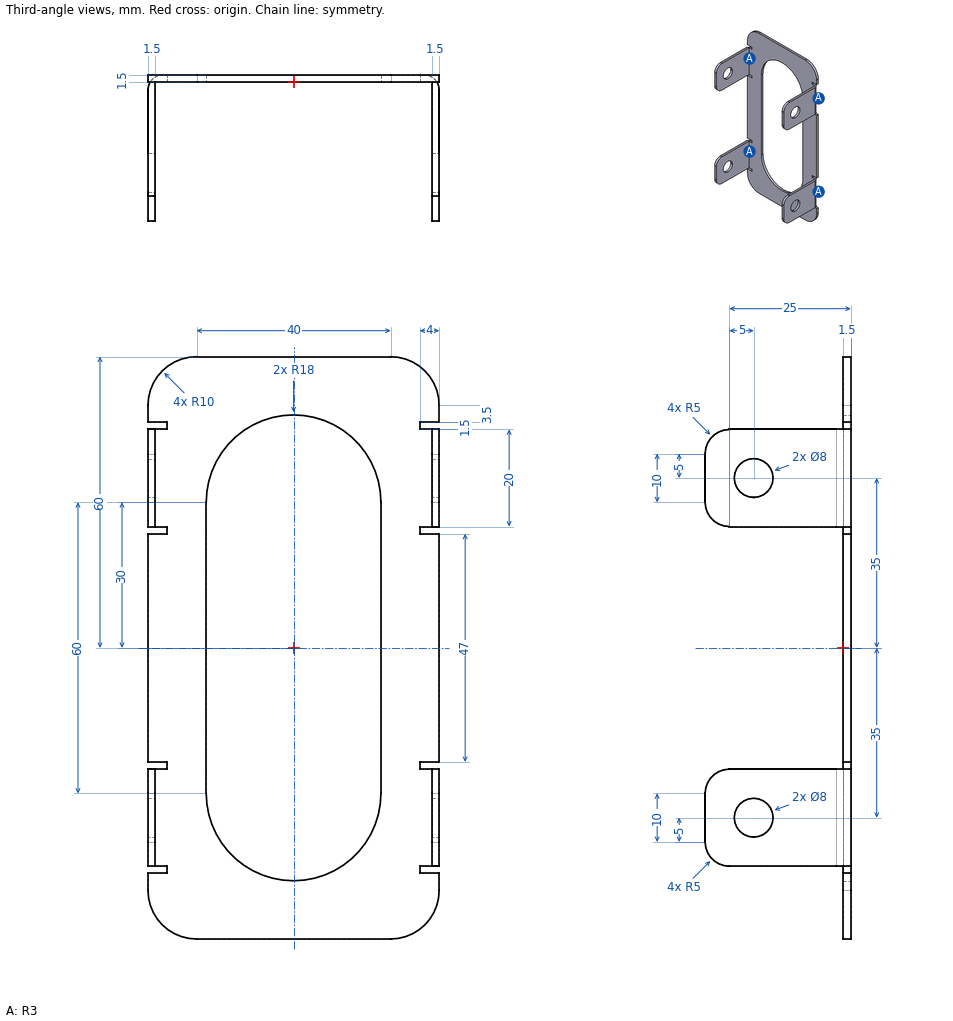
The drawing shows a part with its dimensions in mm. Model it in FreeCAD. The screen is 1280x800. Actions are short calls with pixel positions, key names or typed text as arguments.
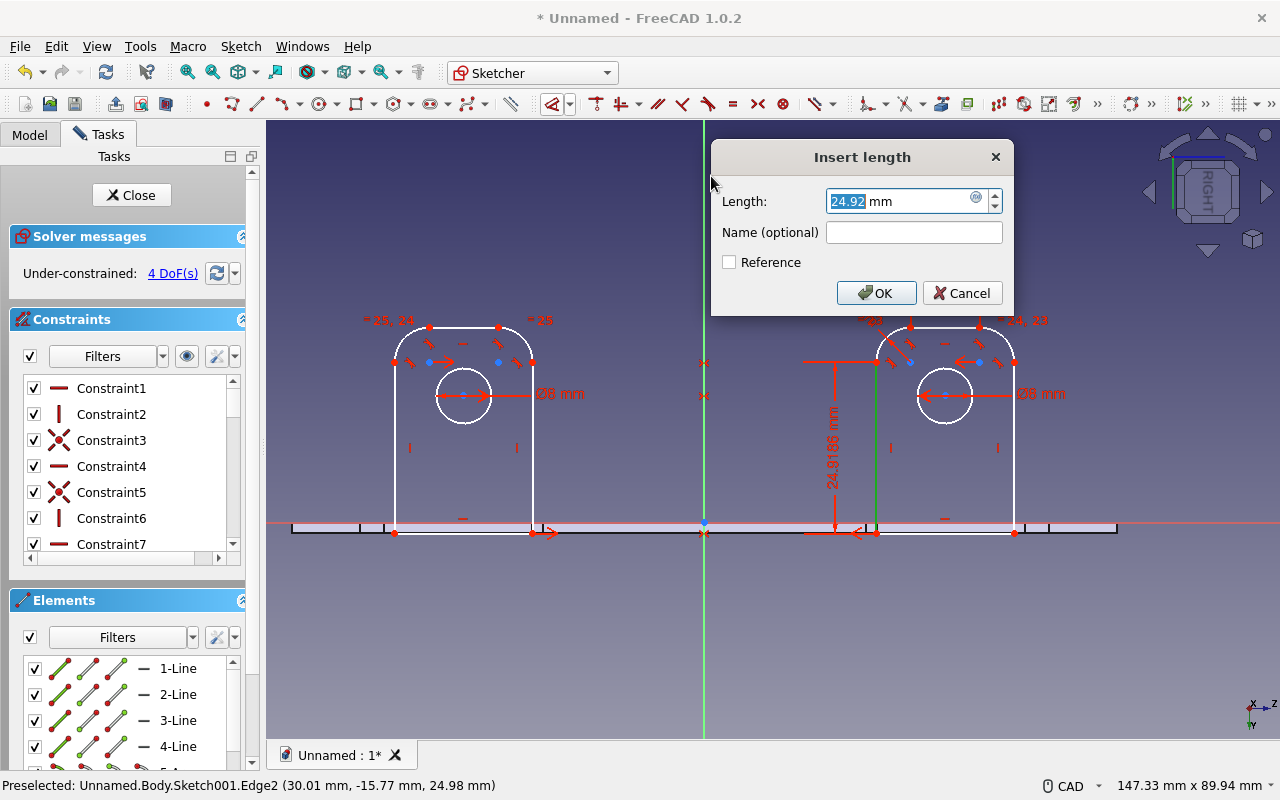
text(25)
key(Return)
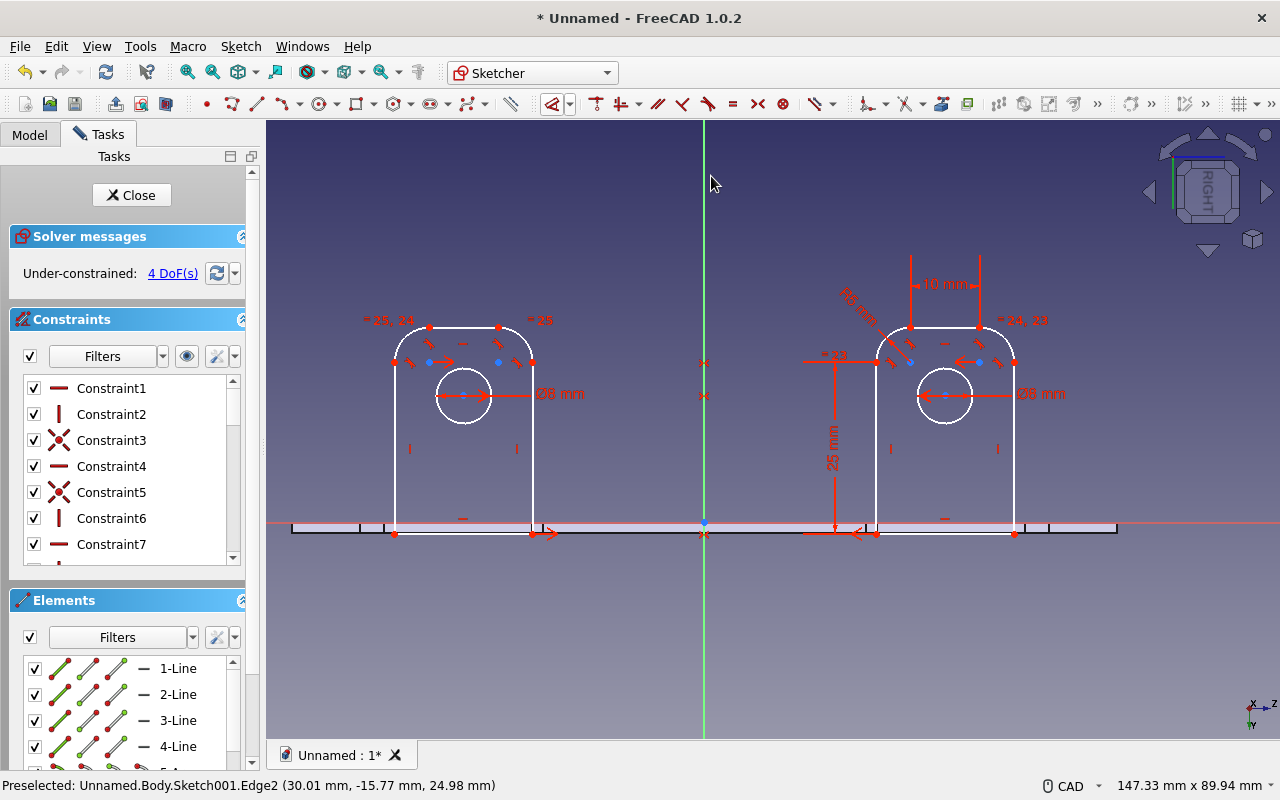
click(945, 396)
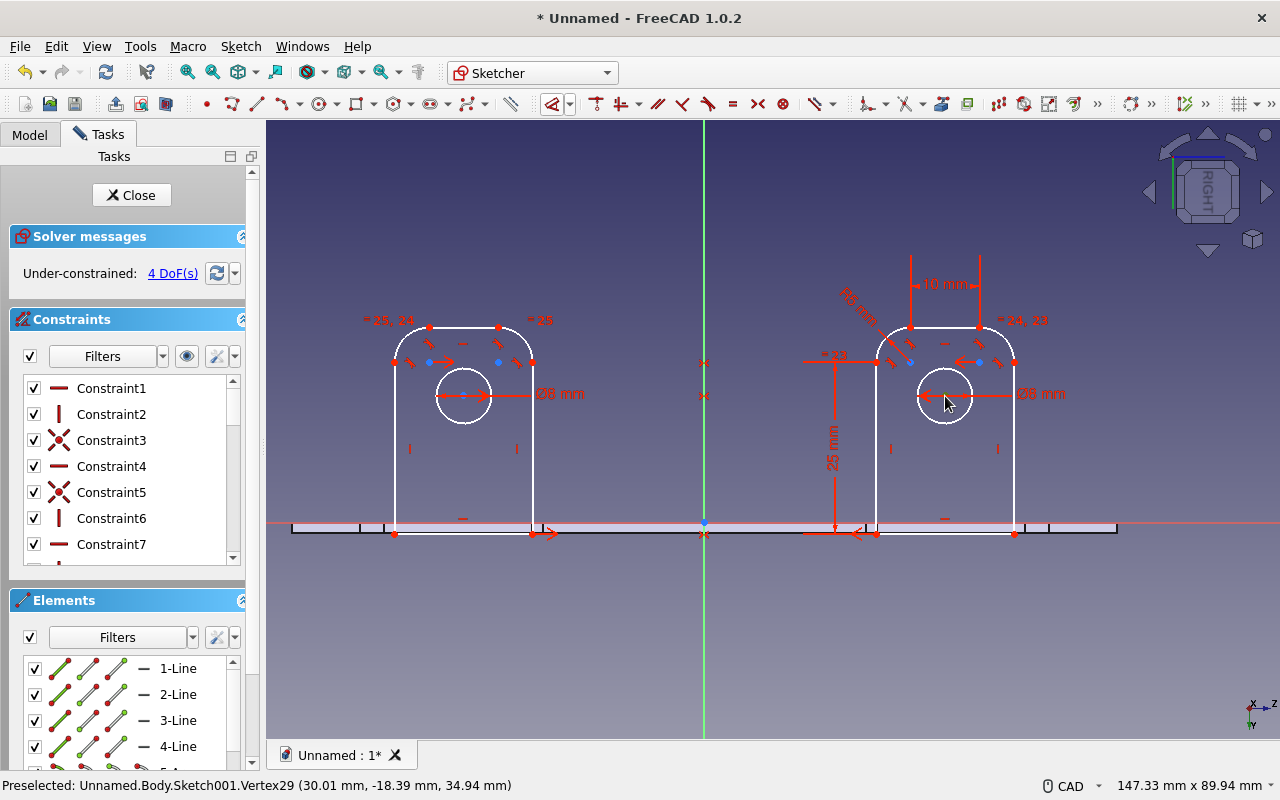
key(l)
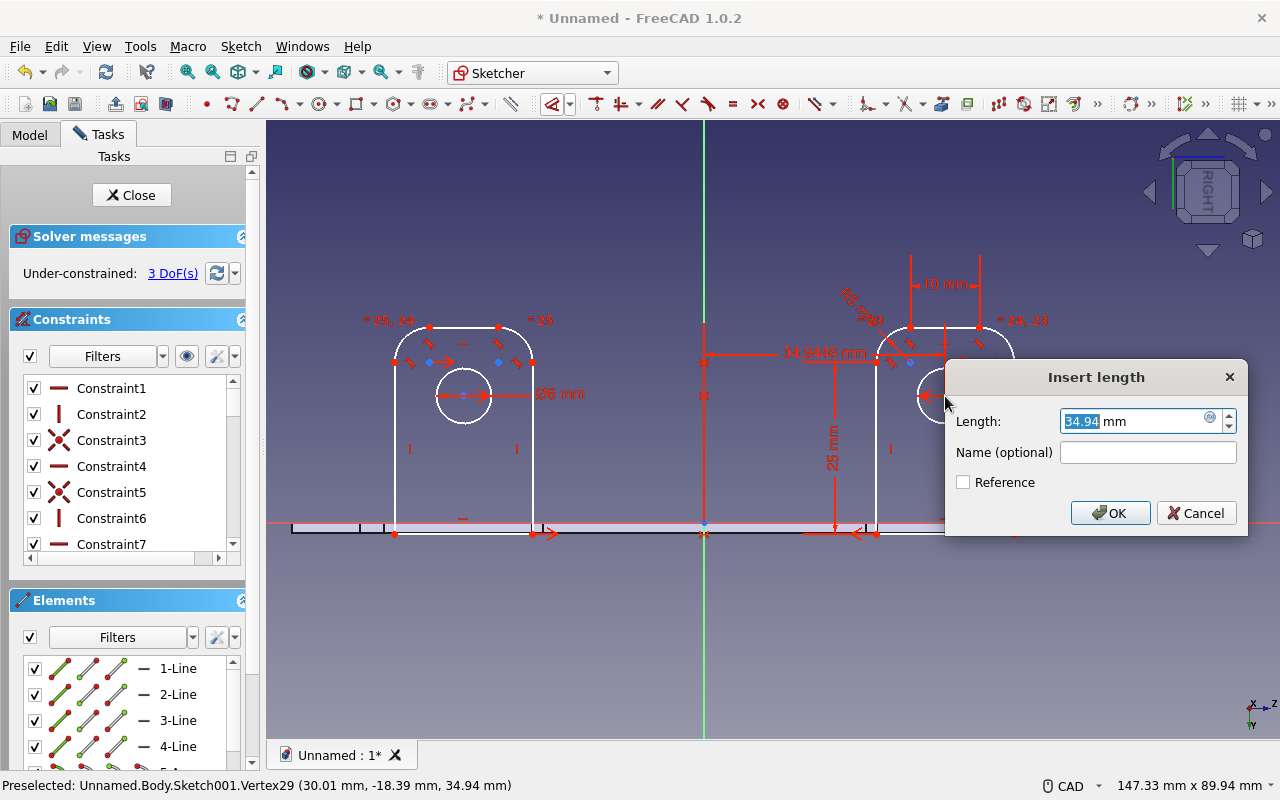
text(35)
key(Return)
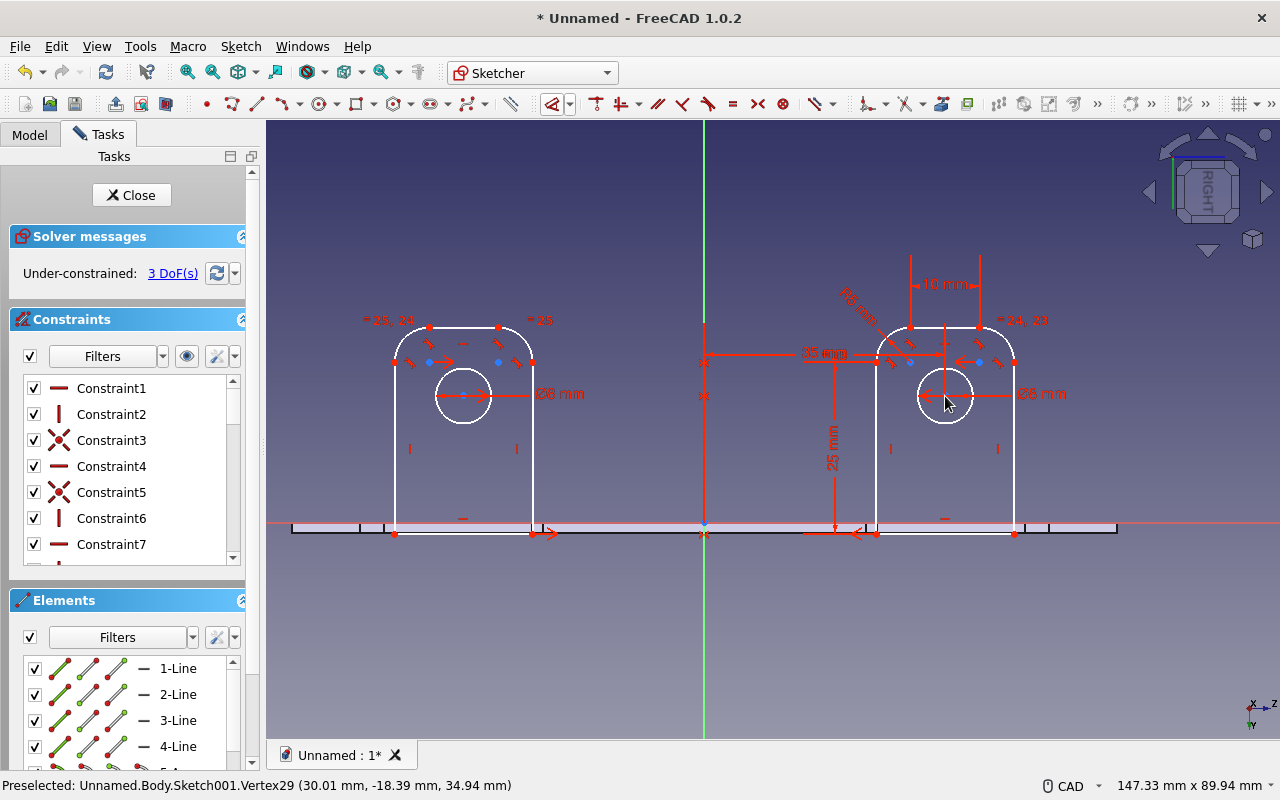
click(980, 328)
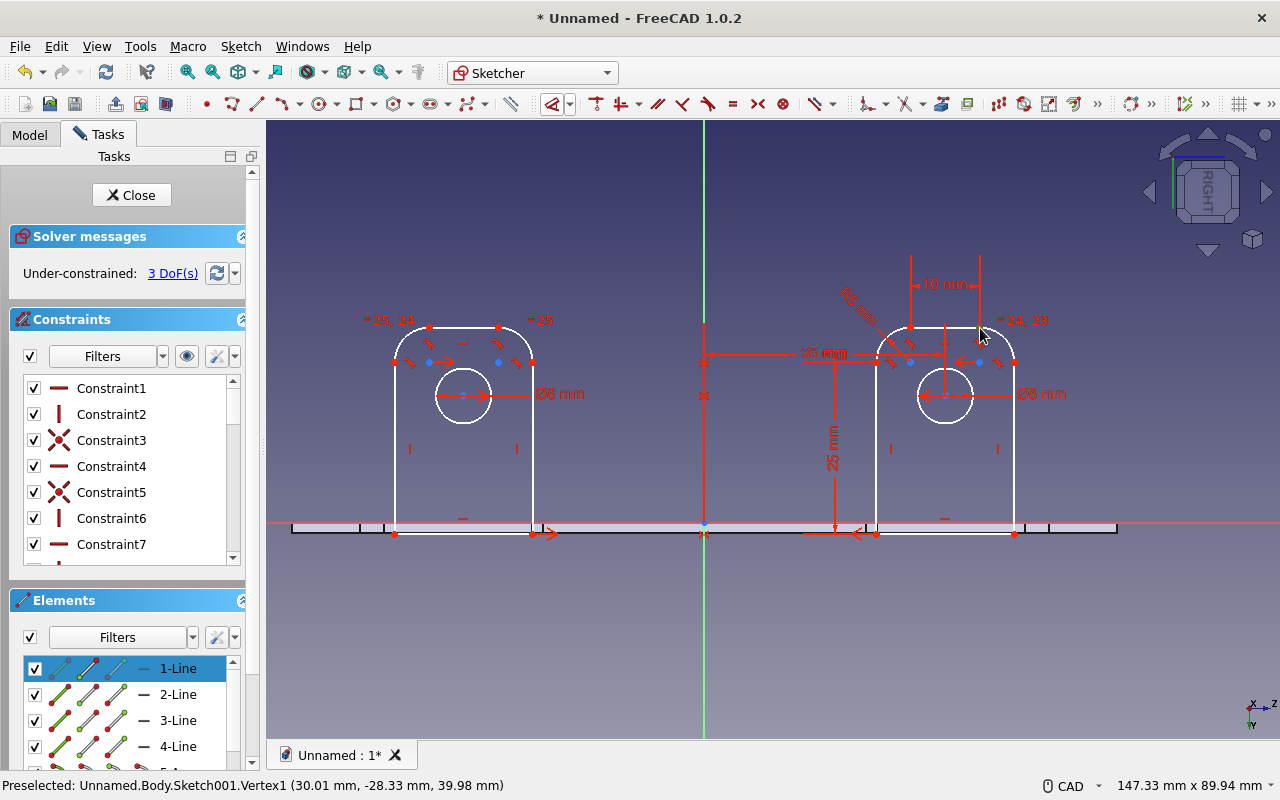
click(945, 396)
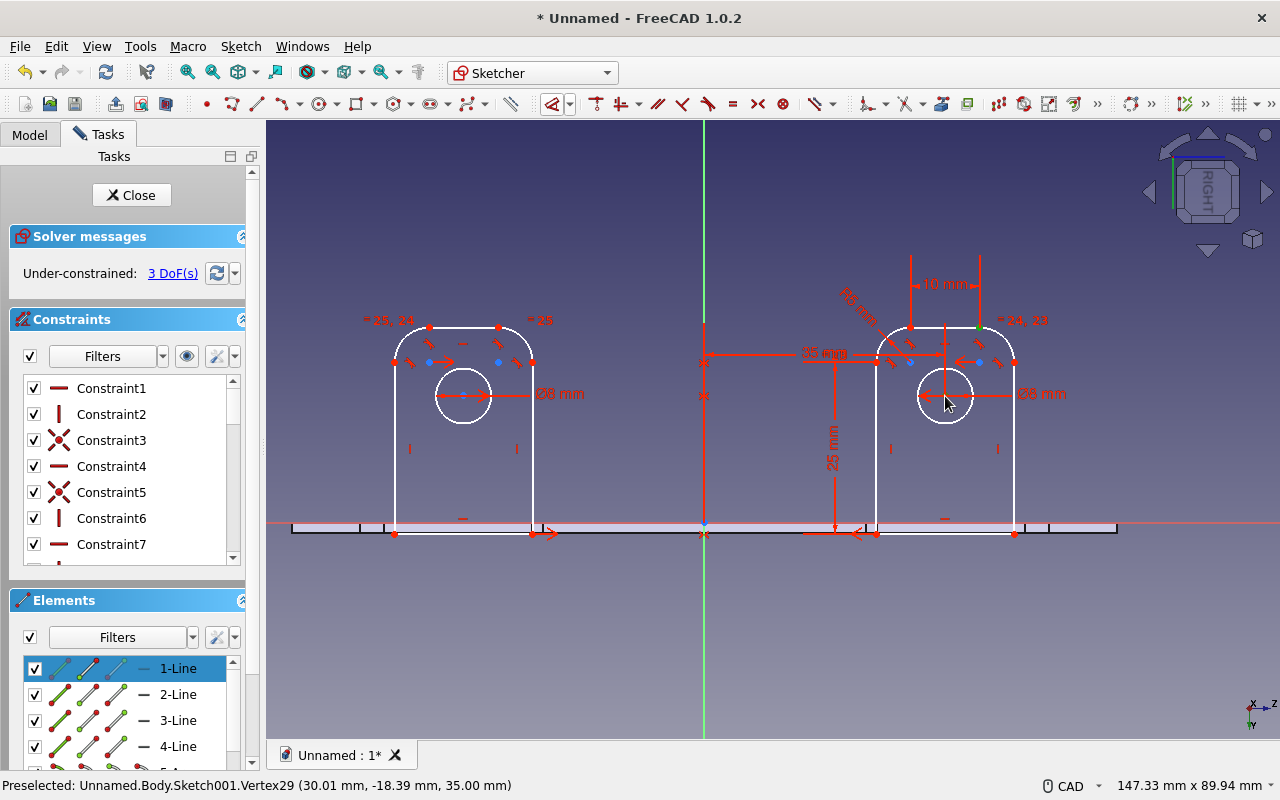
key(l)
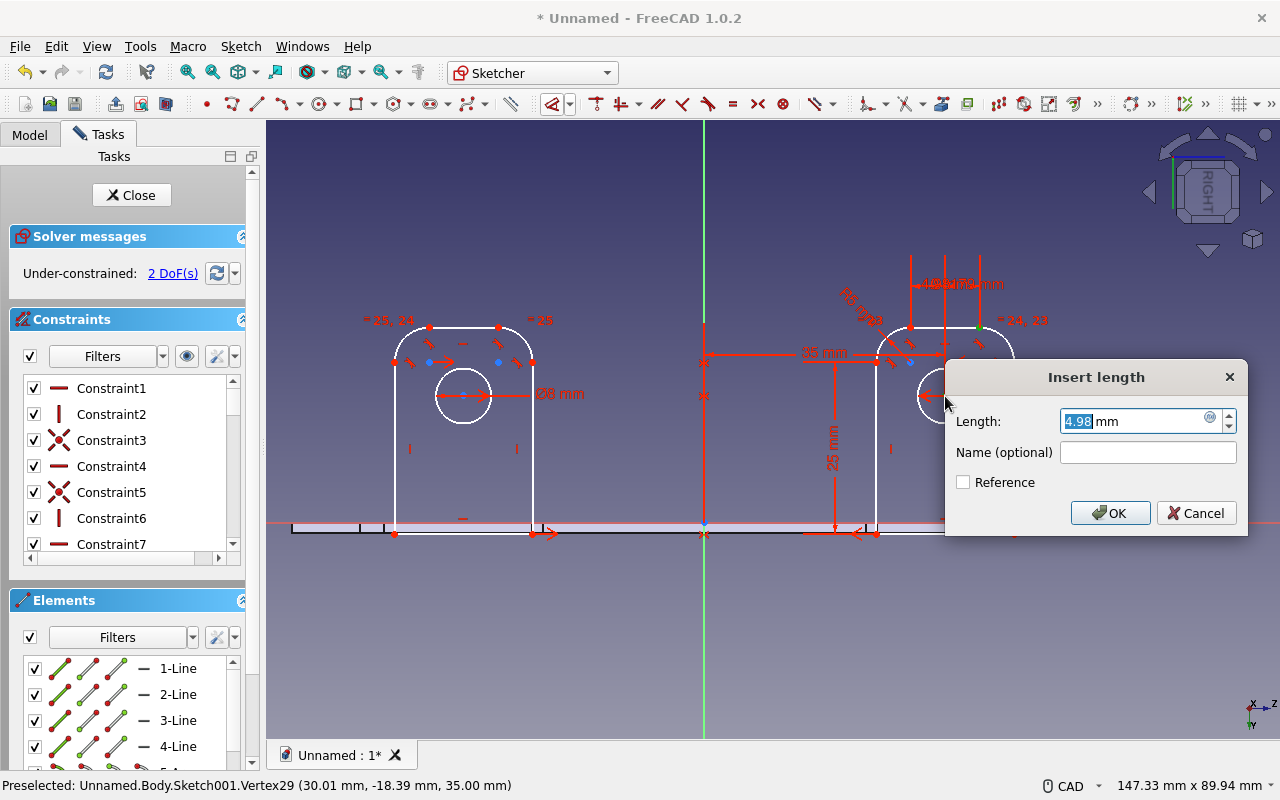
text(5)
key(Return)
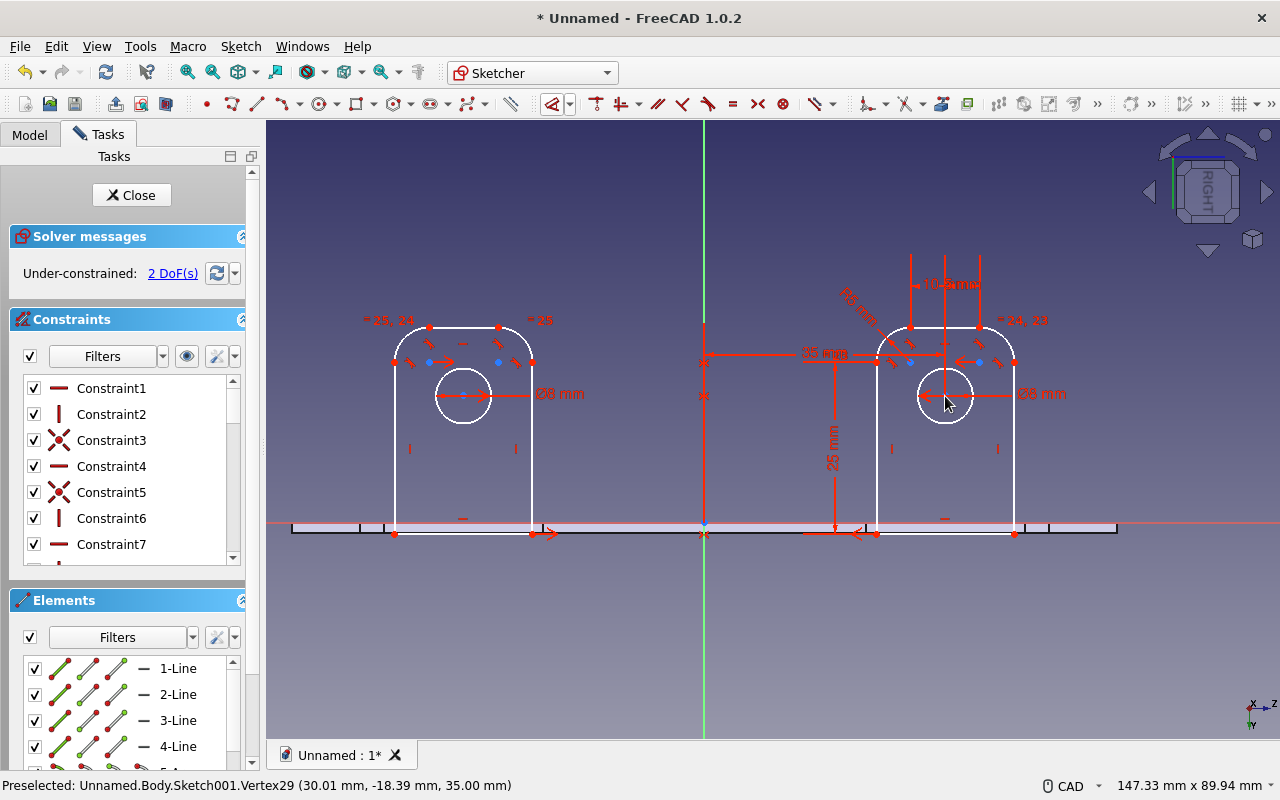
click(877, 362)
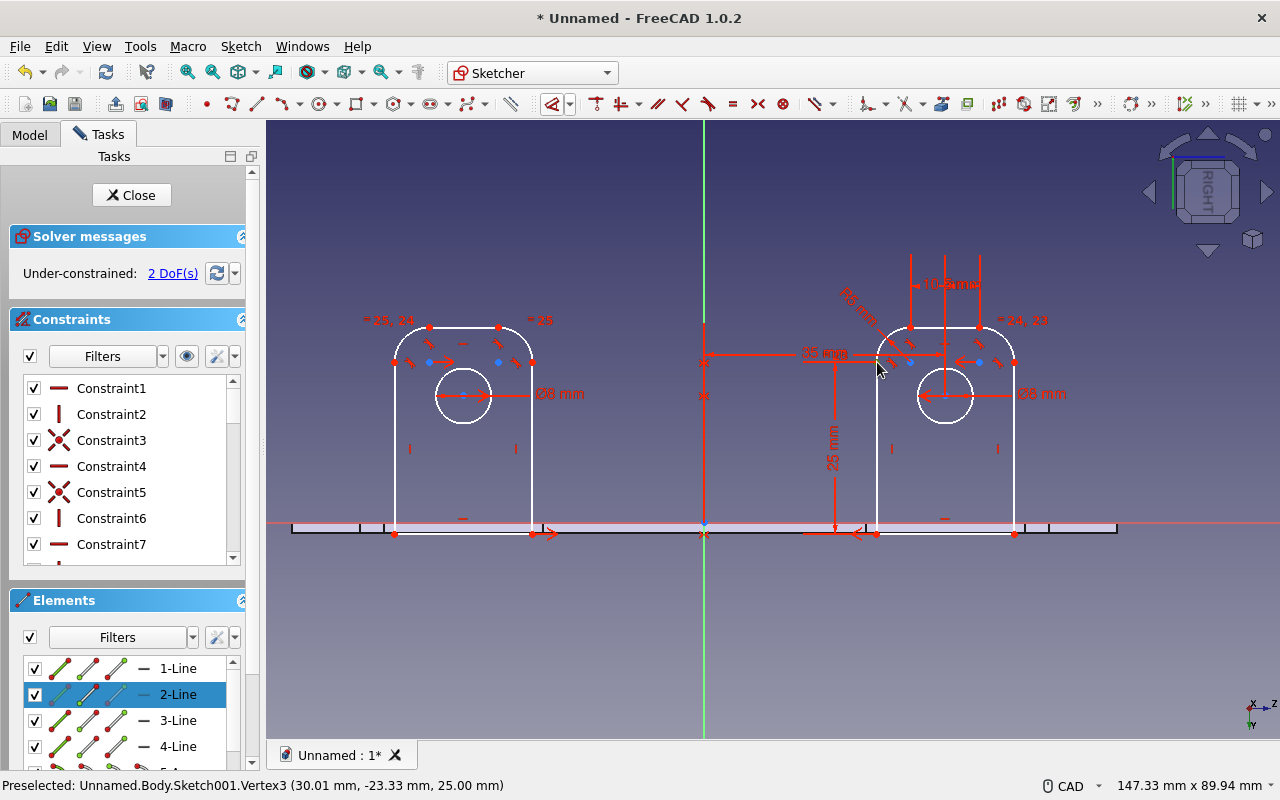
click(945, 396)